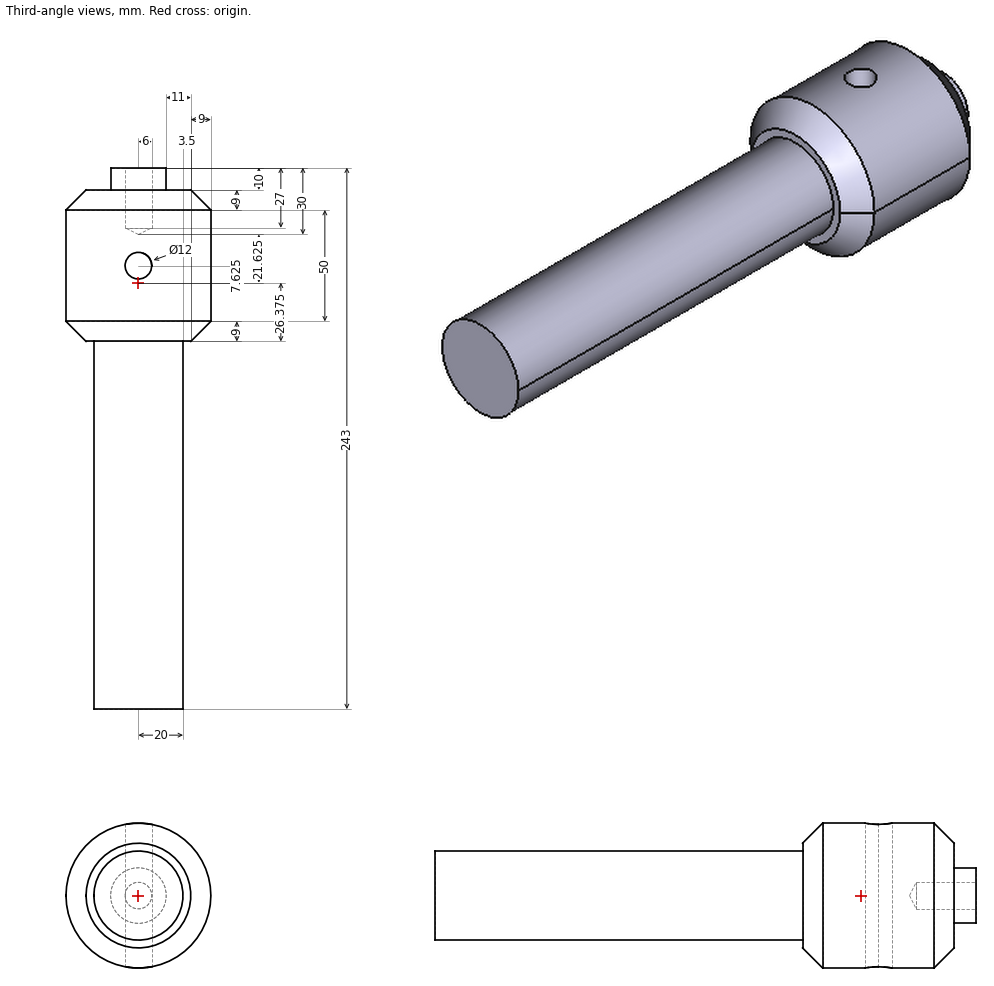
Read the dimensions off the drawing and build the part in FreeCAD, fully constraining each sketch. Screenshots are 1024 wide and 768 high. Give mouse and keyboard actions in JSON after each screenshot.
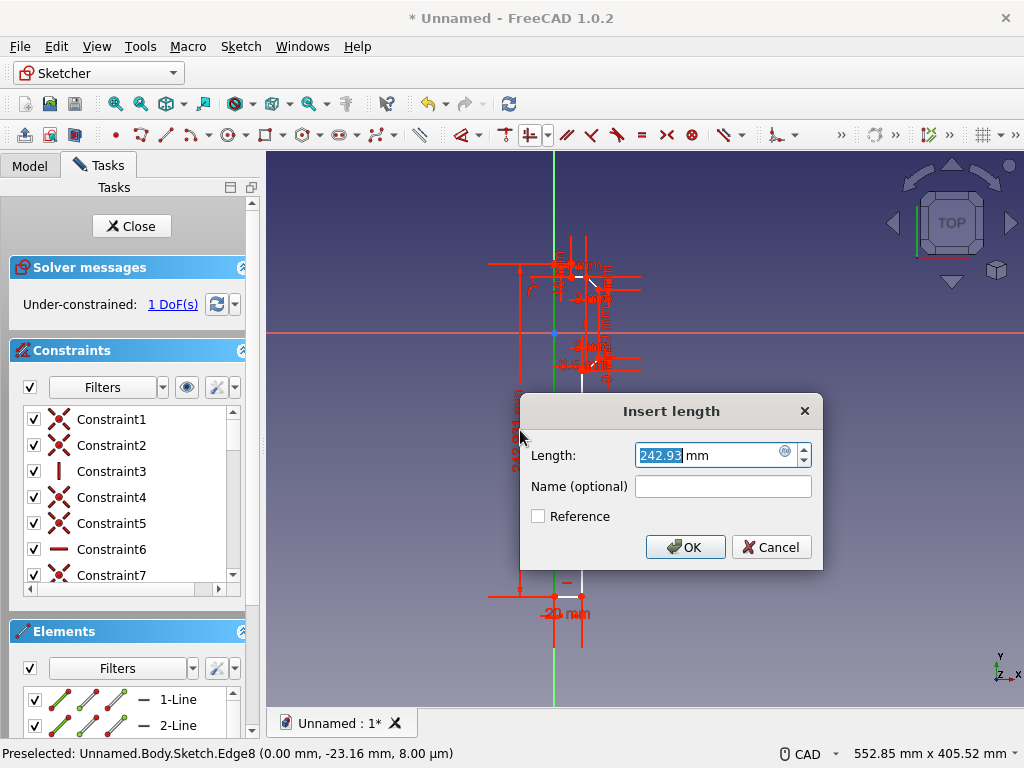
{"action": "type", "text": "243"}
{"action": "key", "text": "Return"}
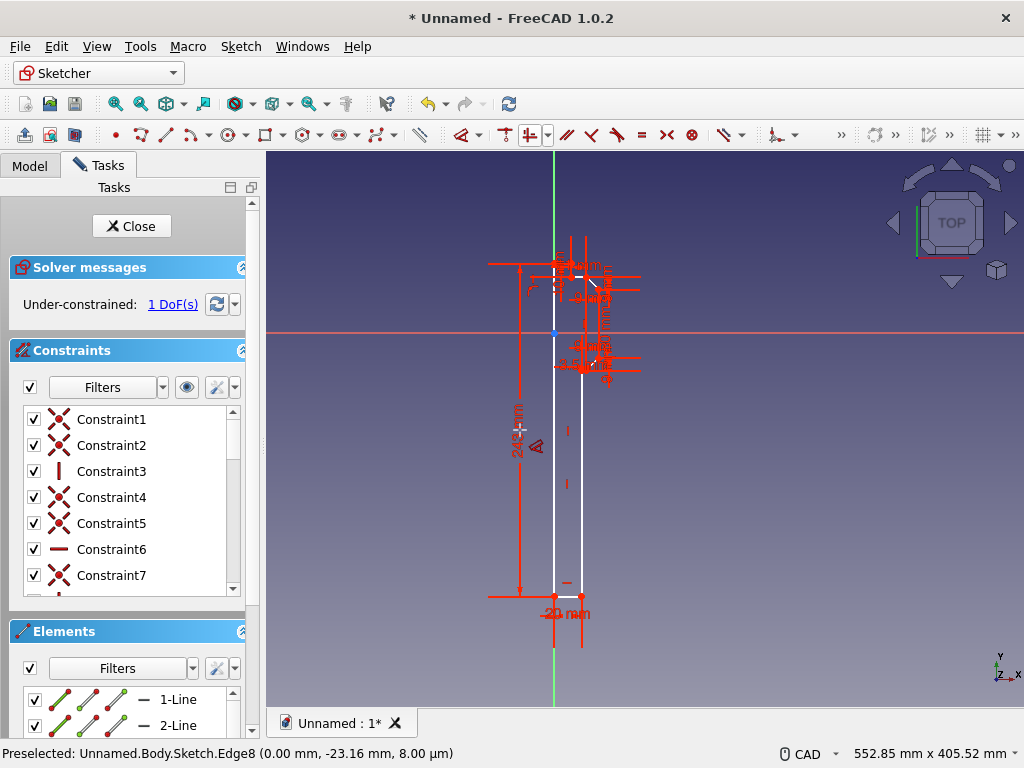
{"action": "scroll", "coordinate": [582, 371], "scroll_direction": "up", "scroll_amount": 5}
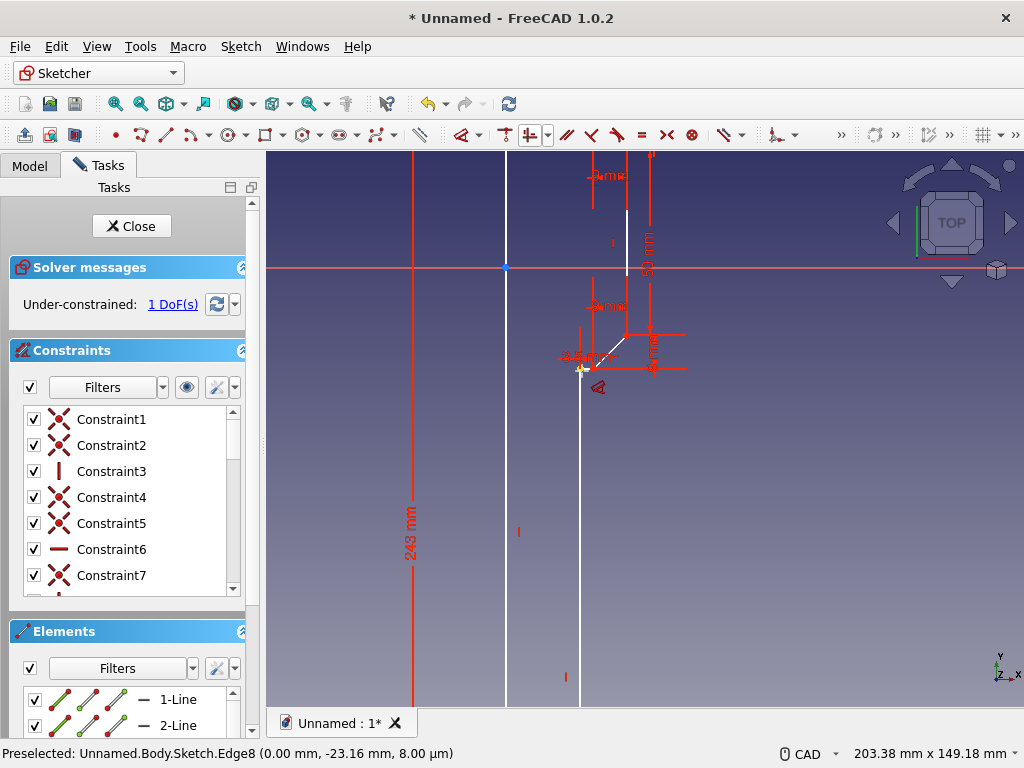
{"action": "left_click", "coordinate": [580, 369]}
{"action": "left_click", "coordinate": [472, 318]}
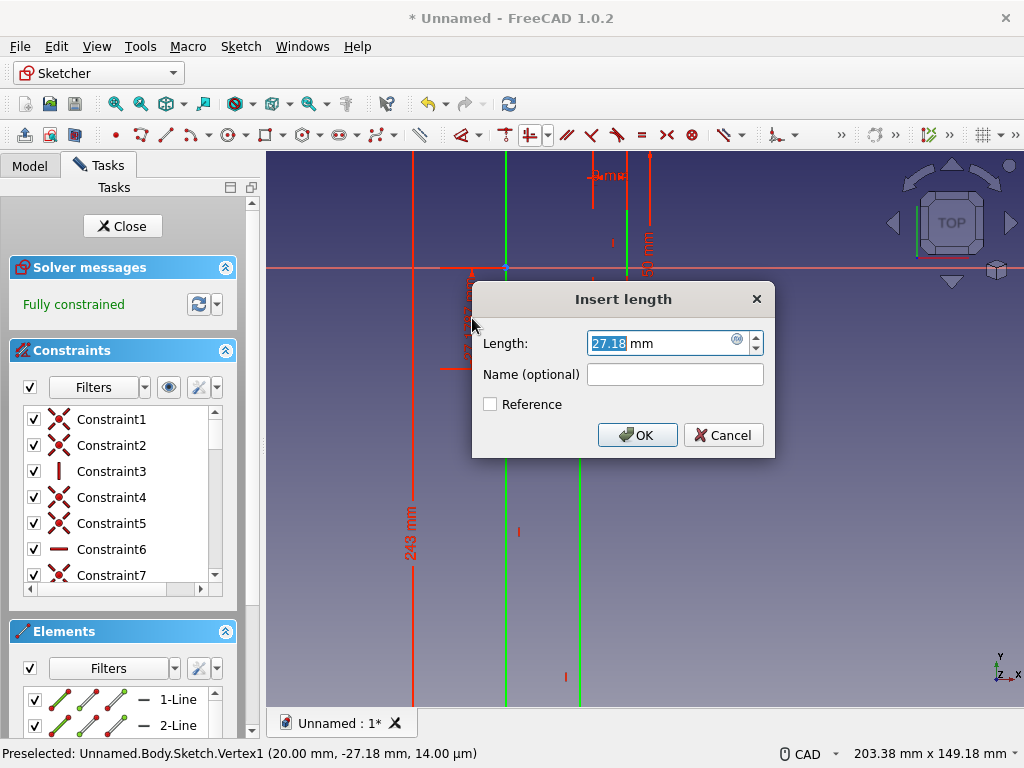
{"action": "type", "text": "26.375"}
{"action": "key", "text": "Return"}
{"action": "key", "text": "Escape"}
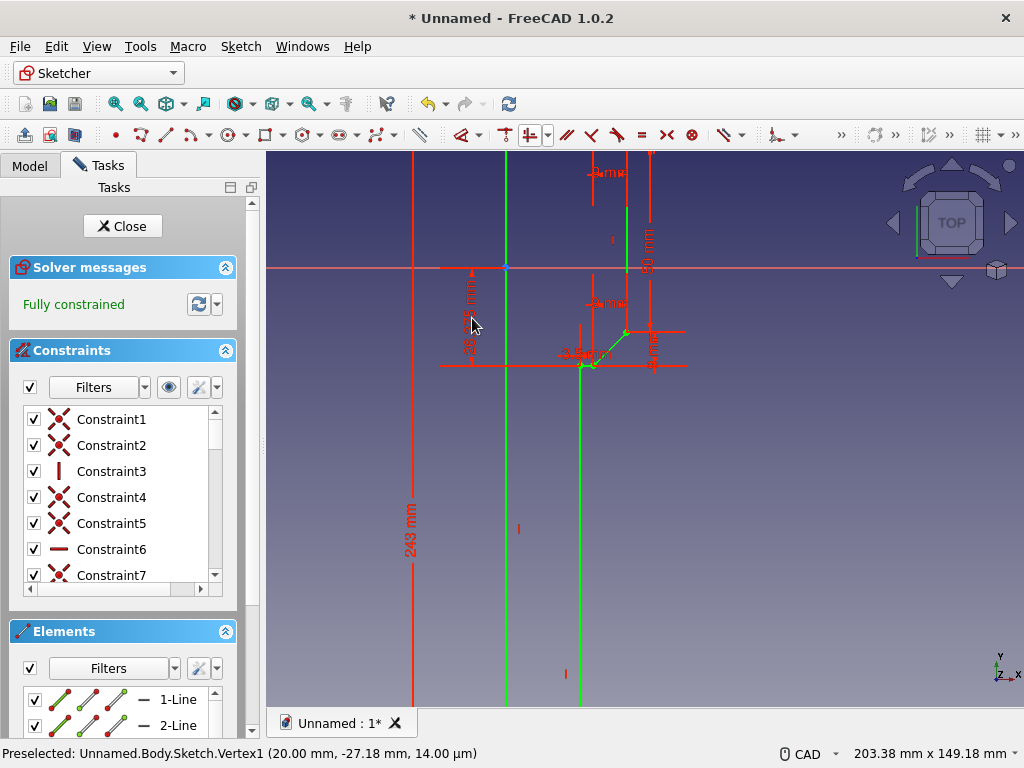
{"action": "left_click", "coordinate": [123, 226]}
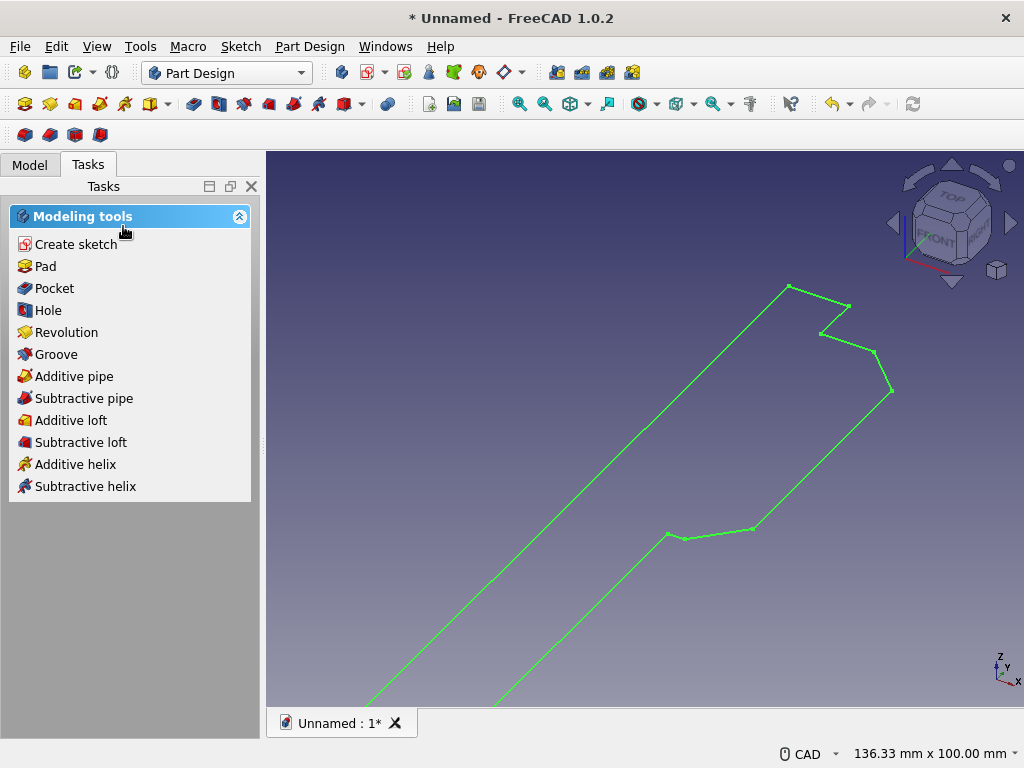
{"action": "left_click", "coordinate": [50, 104]}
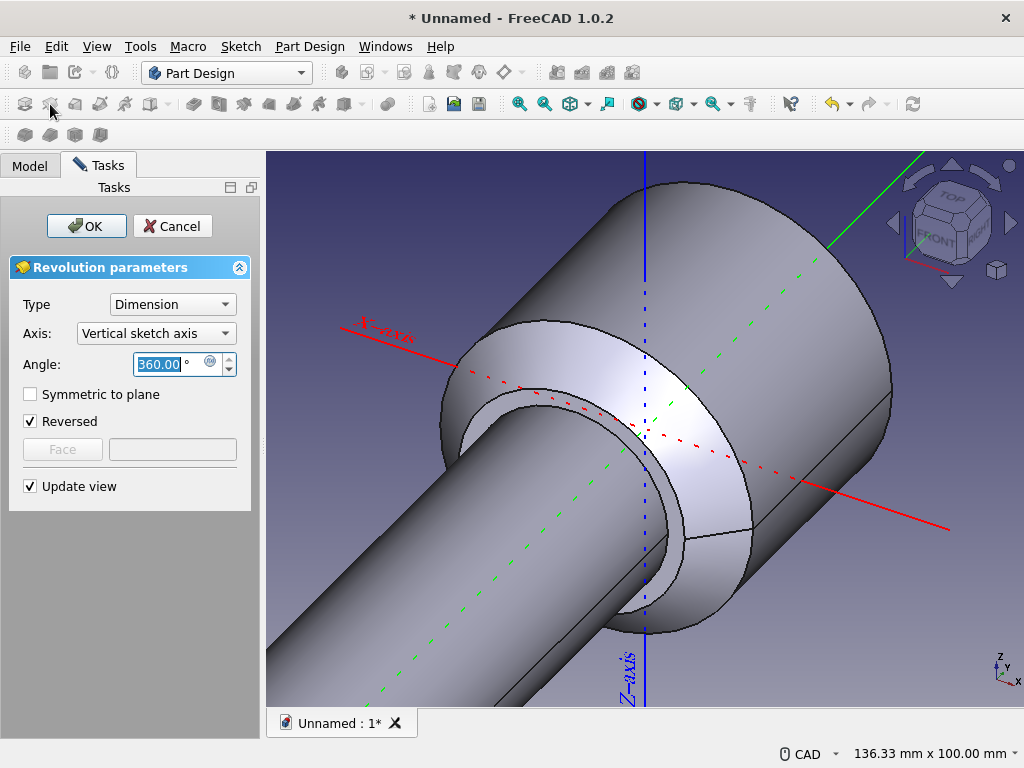
{"action": "left_click", "coordinate": [87, 226]}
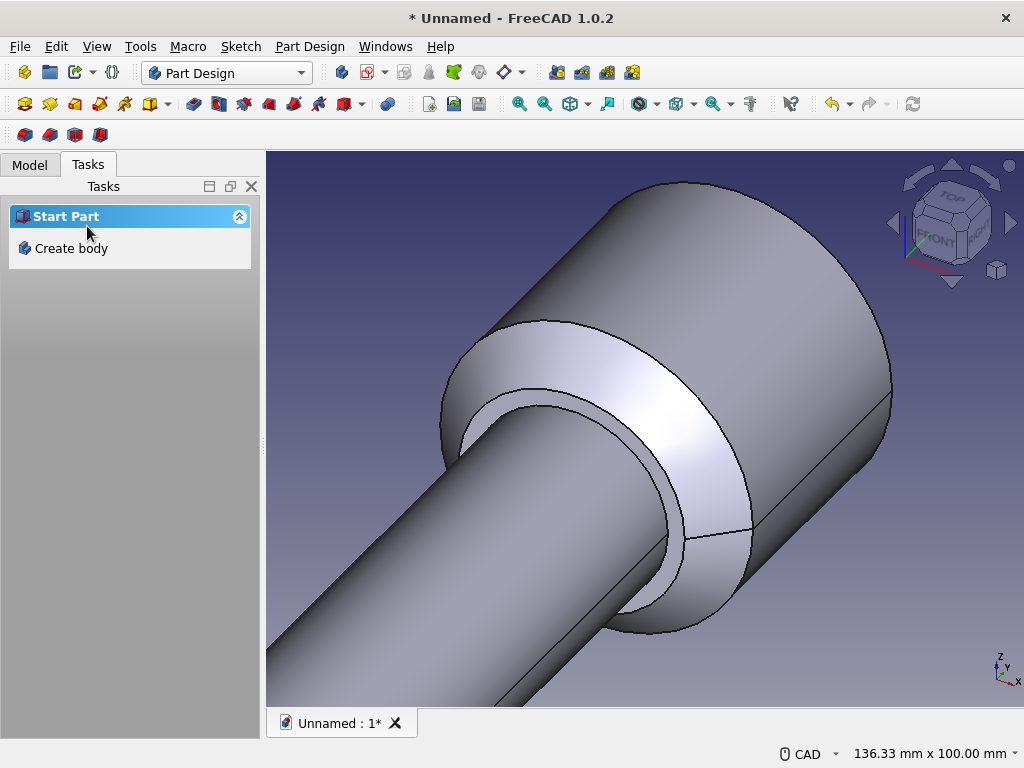
{"action": "key", "text": "v f"}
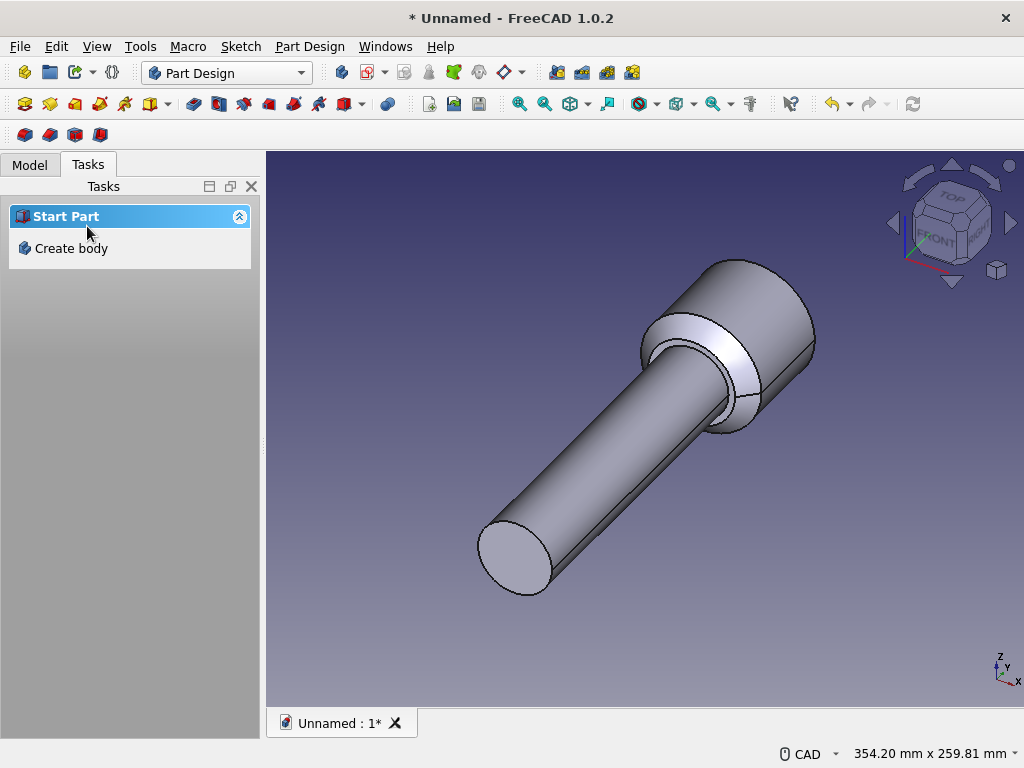
{"action": "left_click", "coordinate": [366, 72]}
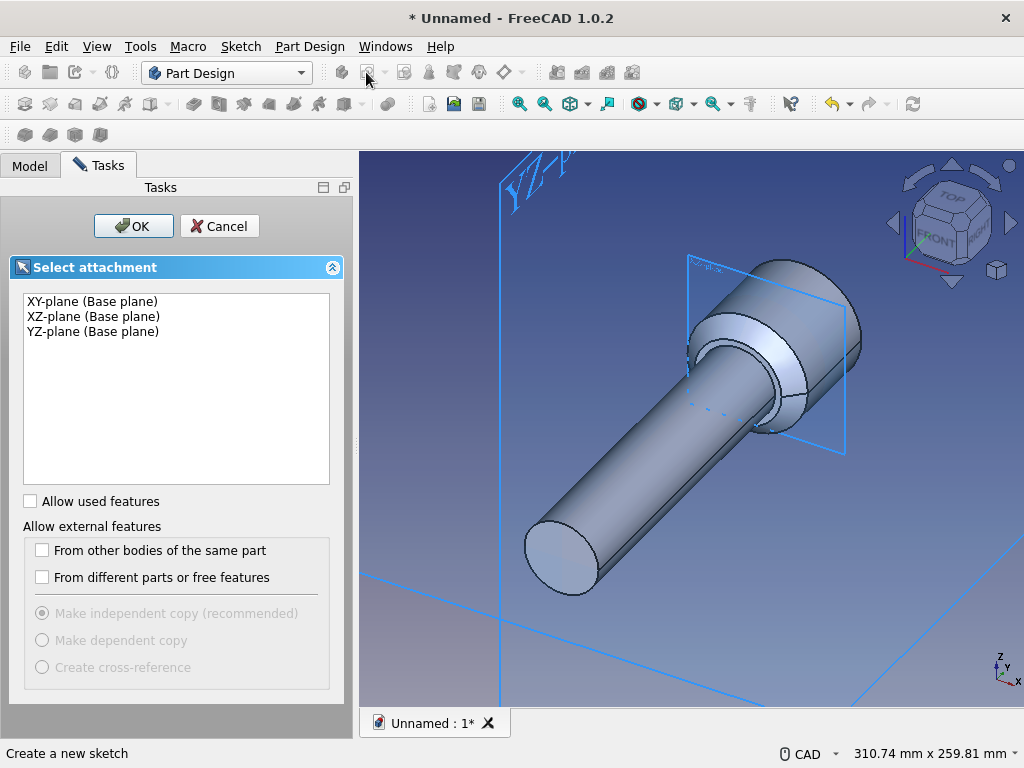
{"action": "left_click", "coordinate": [84, 302]}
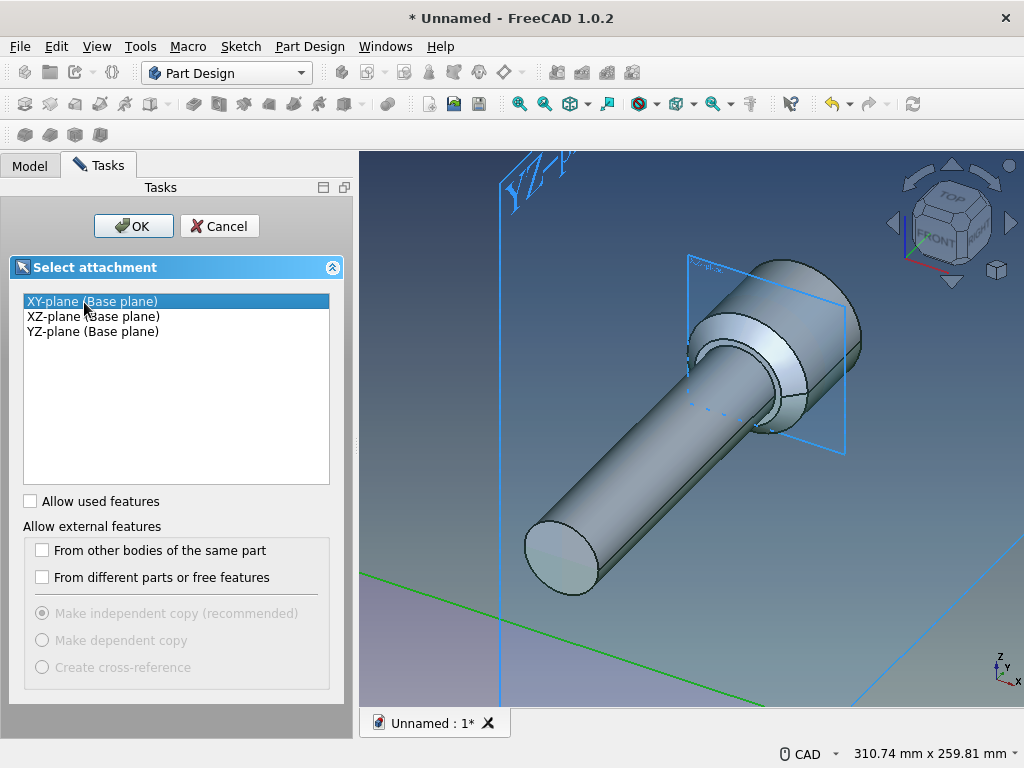
{"action": "left_click", "coordinate": [134, 226]}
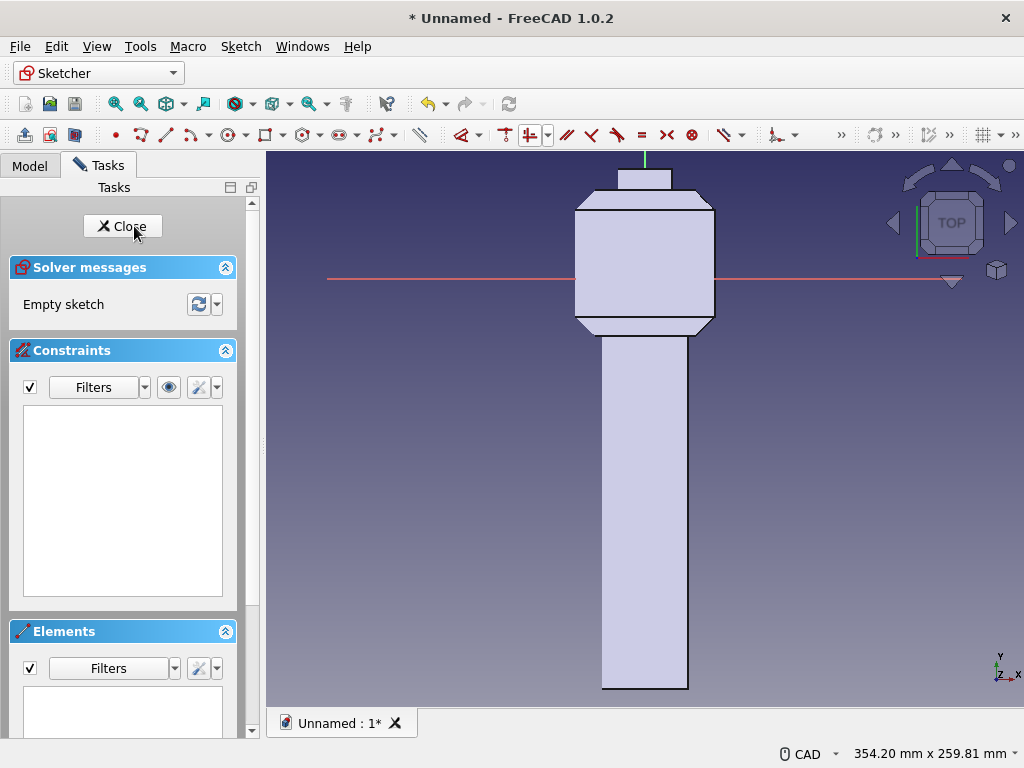
{"action": "key", "text": "q s"}